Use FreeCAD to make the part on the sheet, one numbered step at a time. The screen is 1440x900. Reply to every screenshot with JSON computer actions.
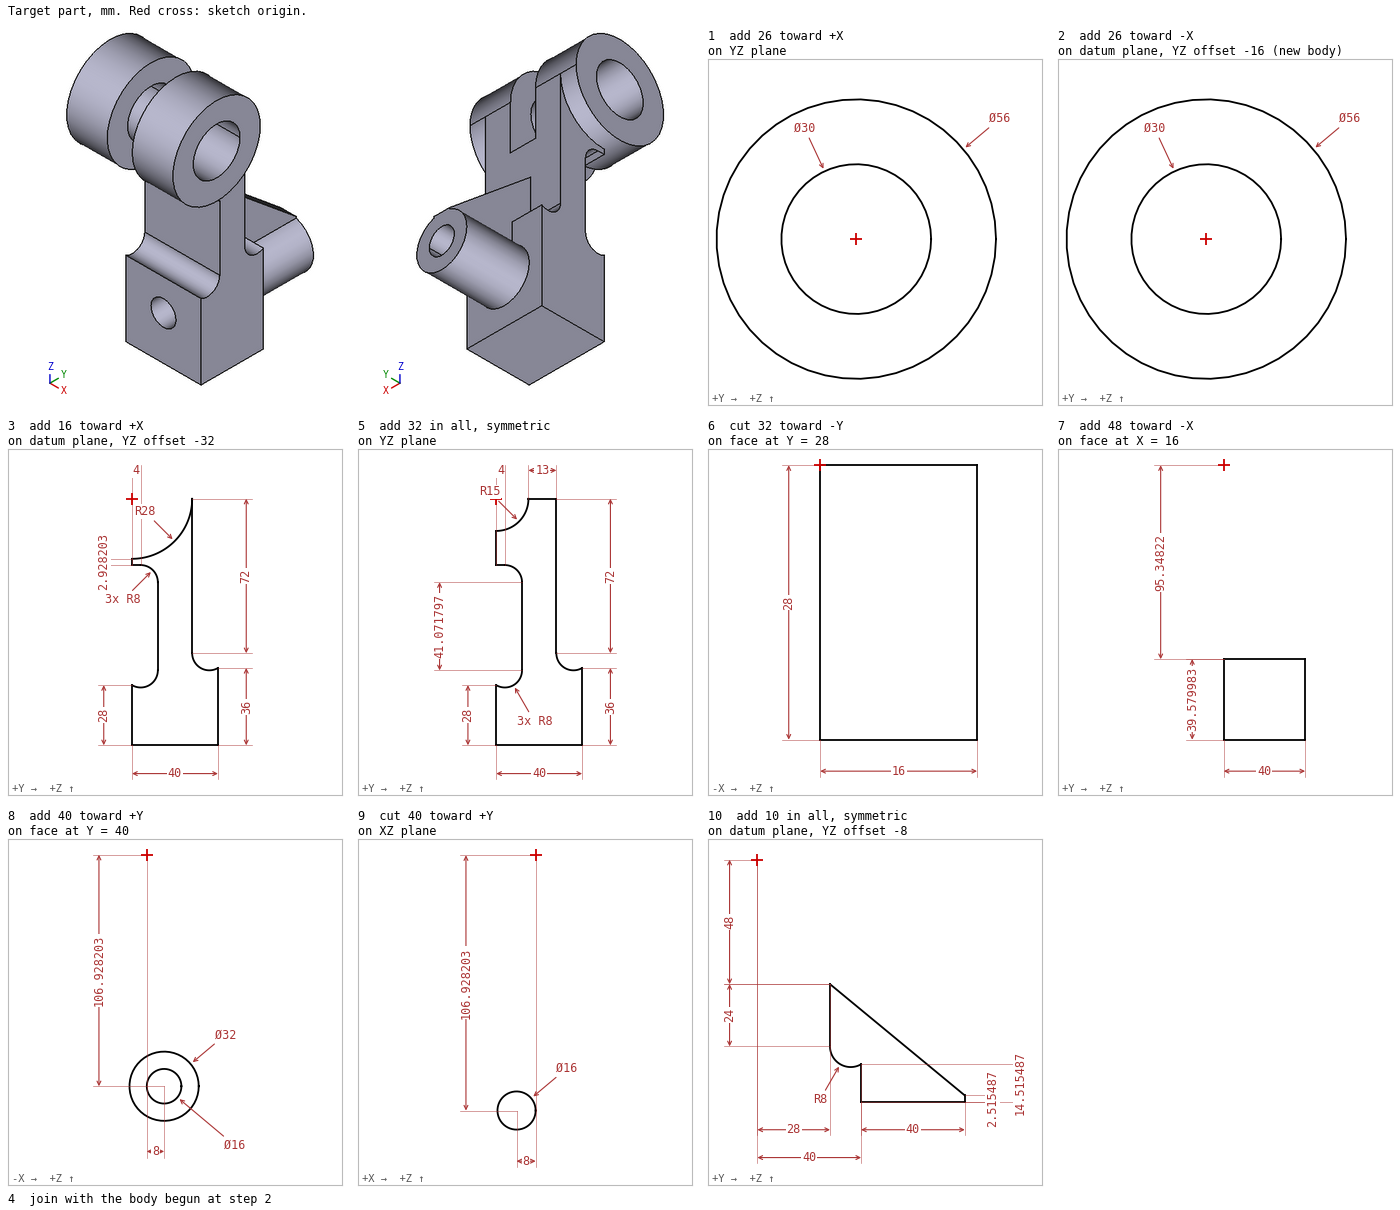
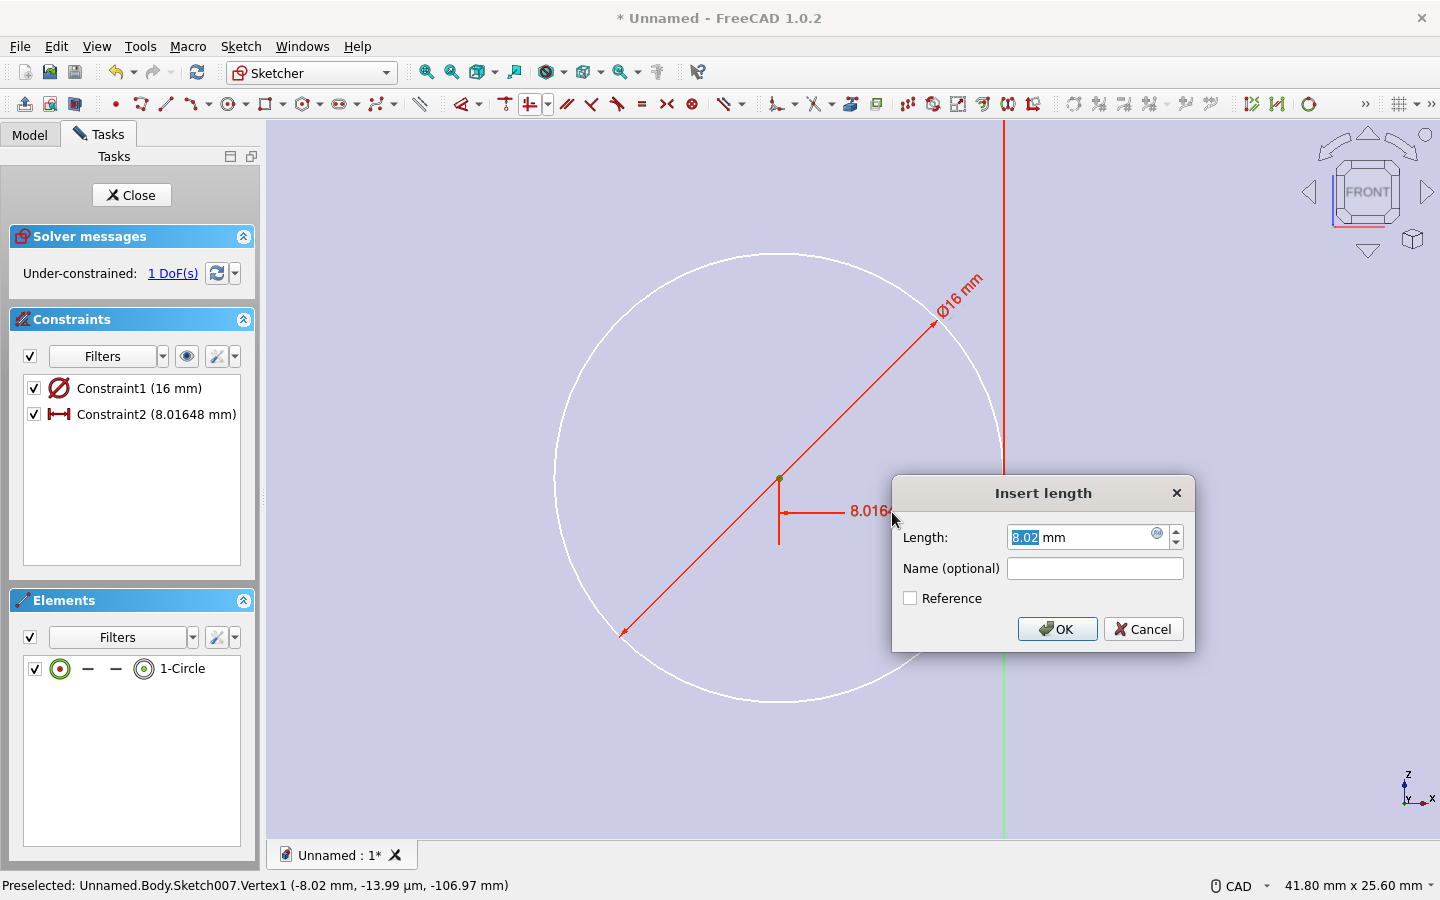
{"action": "type", "text": "8"}
{"action": "key", "text": "Return"}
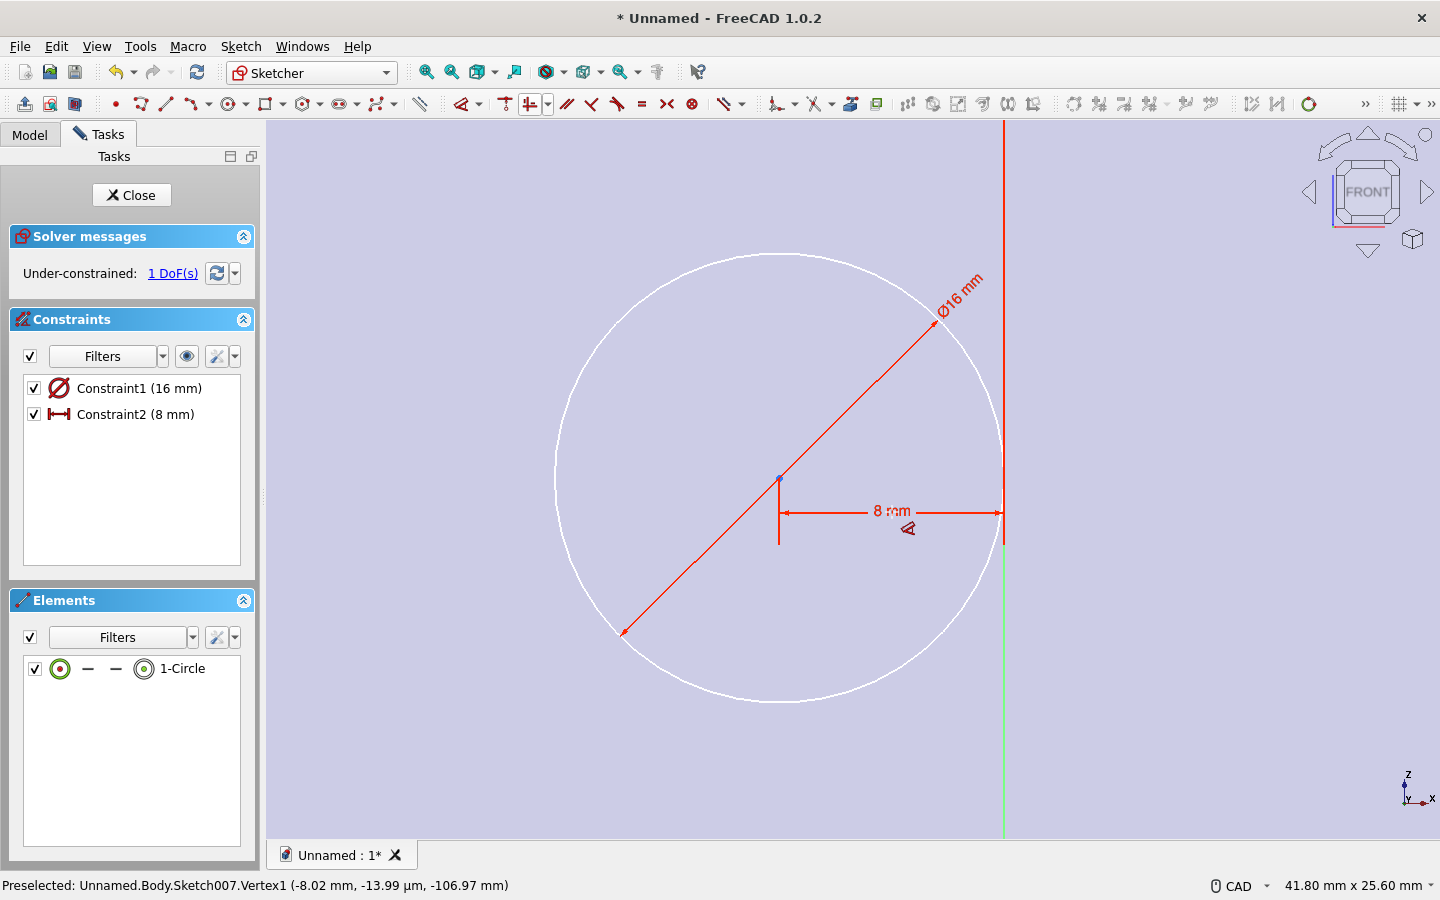
{"action": "left_click", "coordinate": [779, 478]}
{"action": "left_click", "coordinate": [1038, 313]}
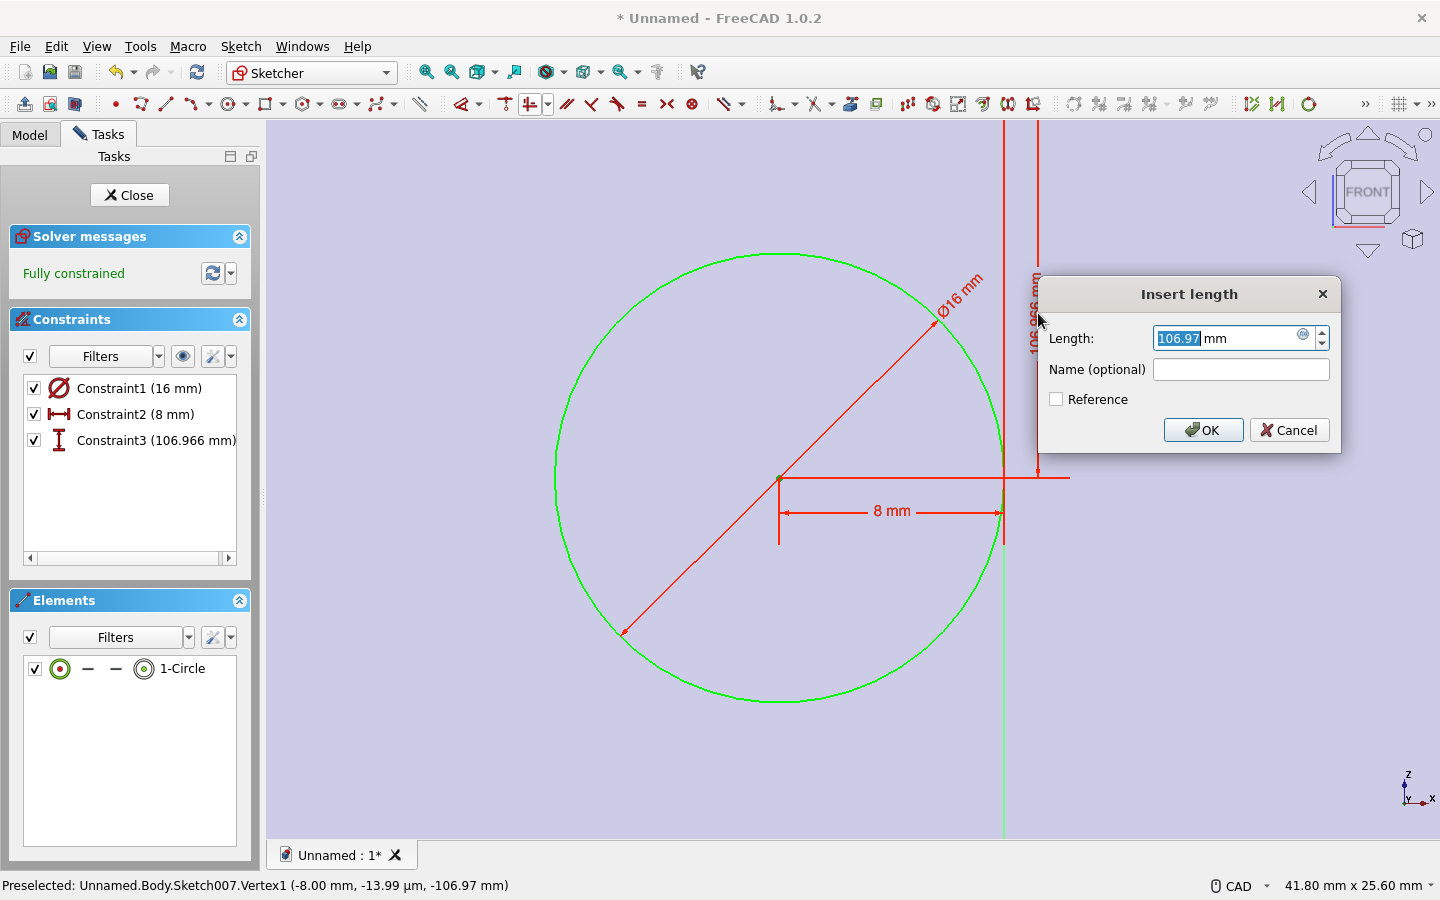
{"action": "type", "text": "106.928203"}
{"action": "key", "text": "Return"}
{"action": "key", "text": "Escape"}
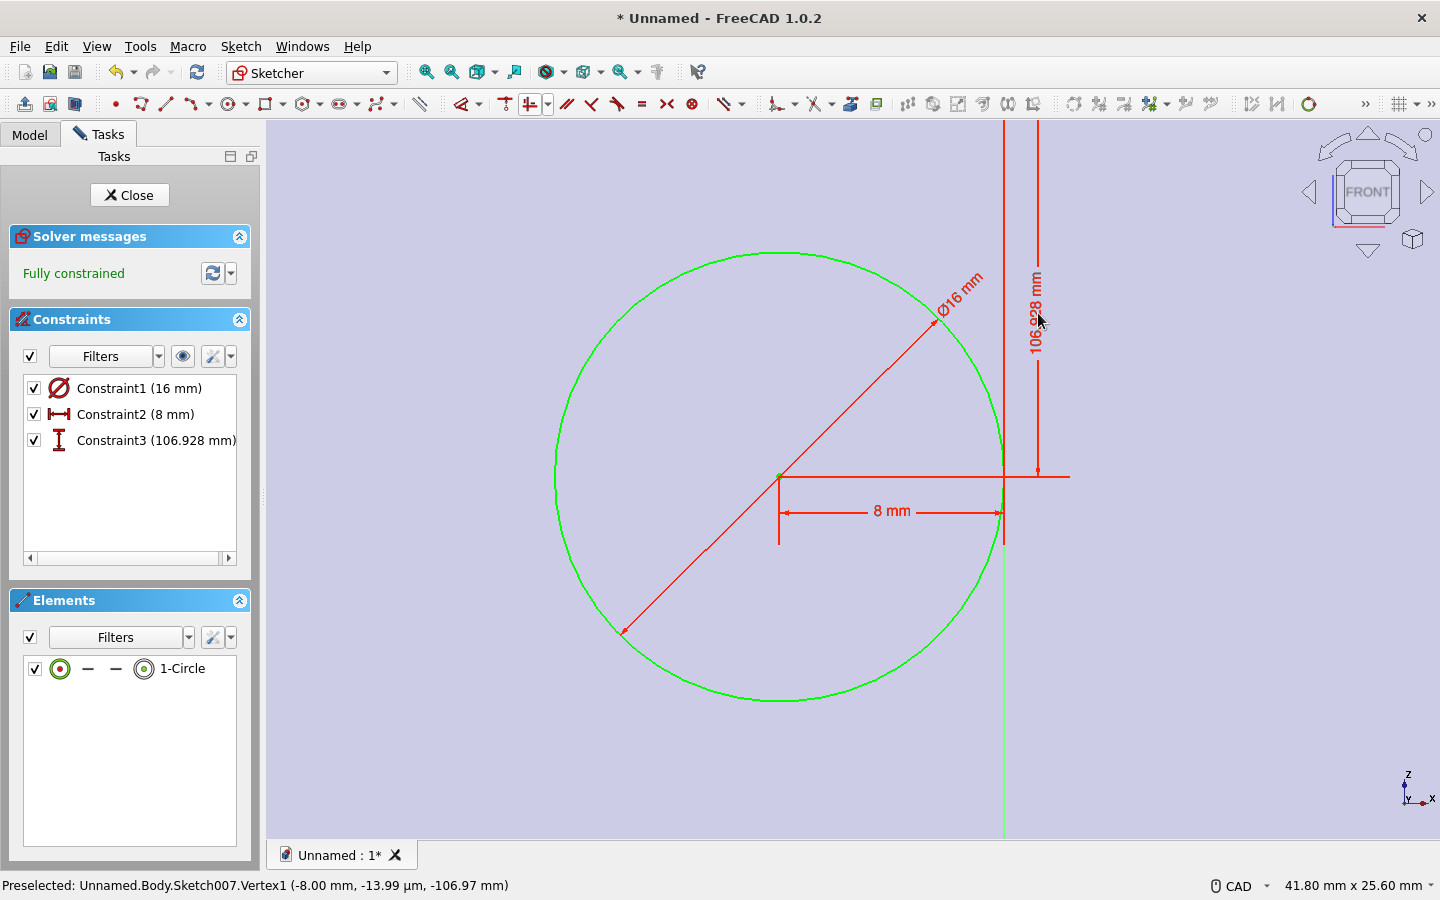
{"action": "left_click", "coordinate": [130, 195]}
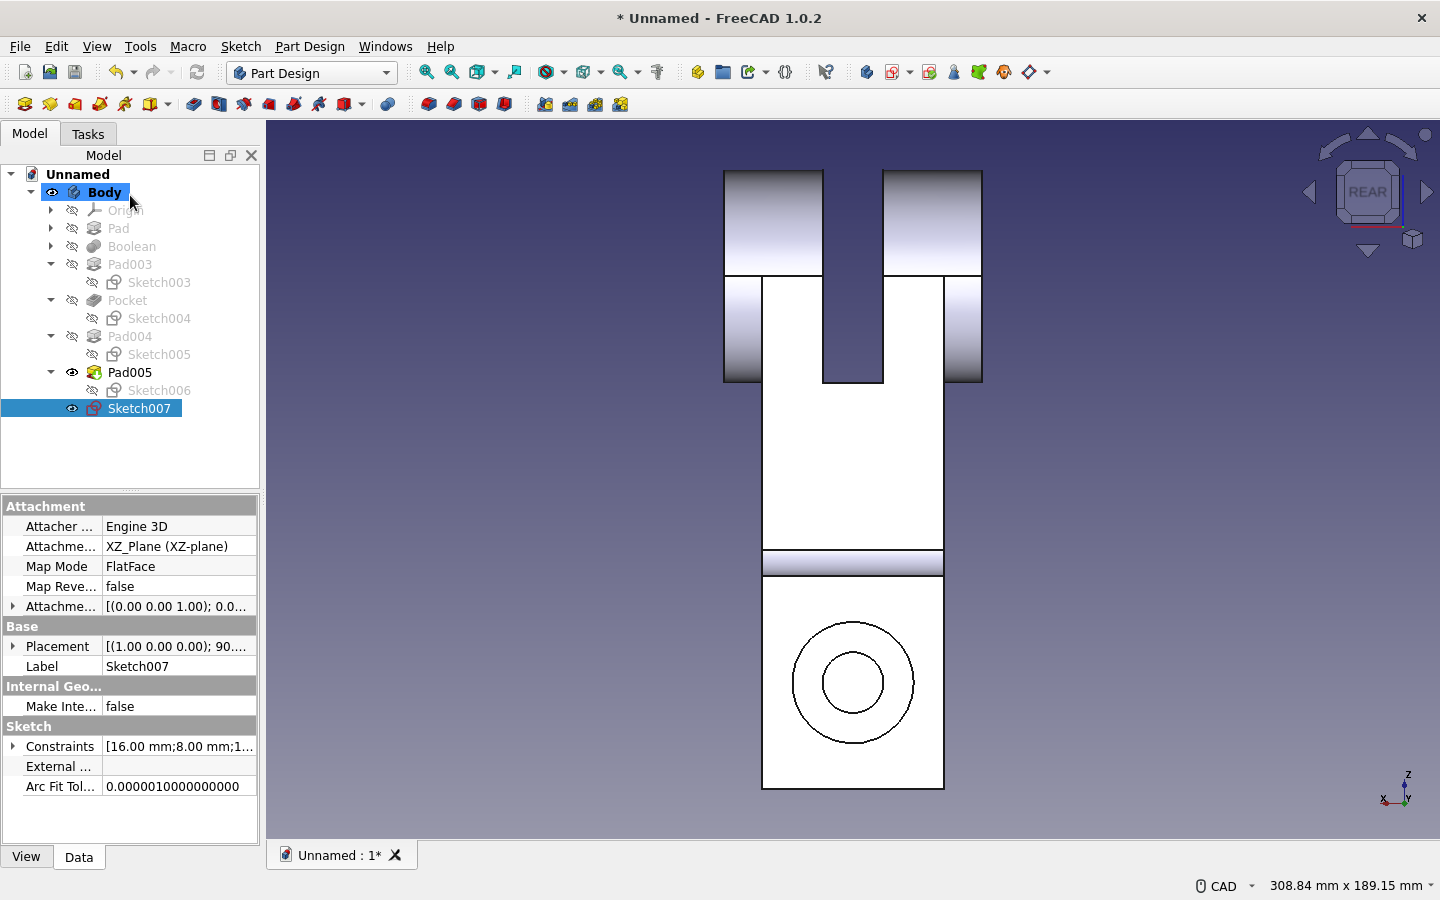
{"action": "left_click", "coordinate": [194, 104]}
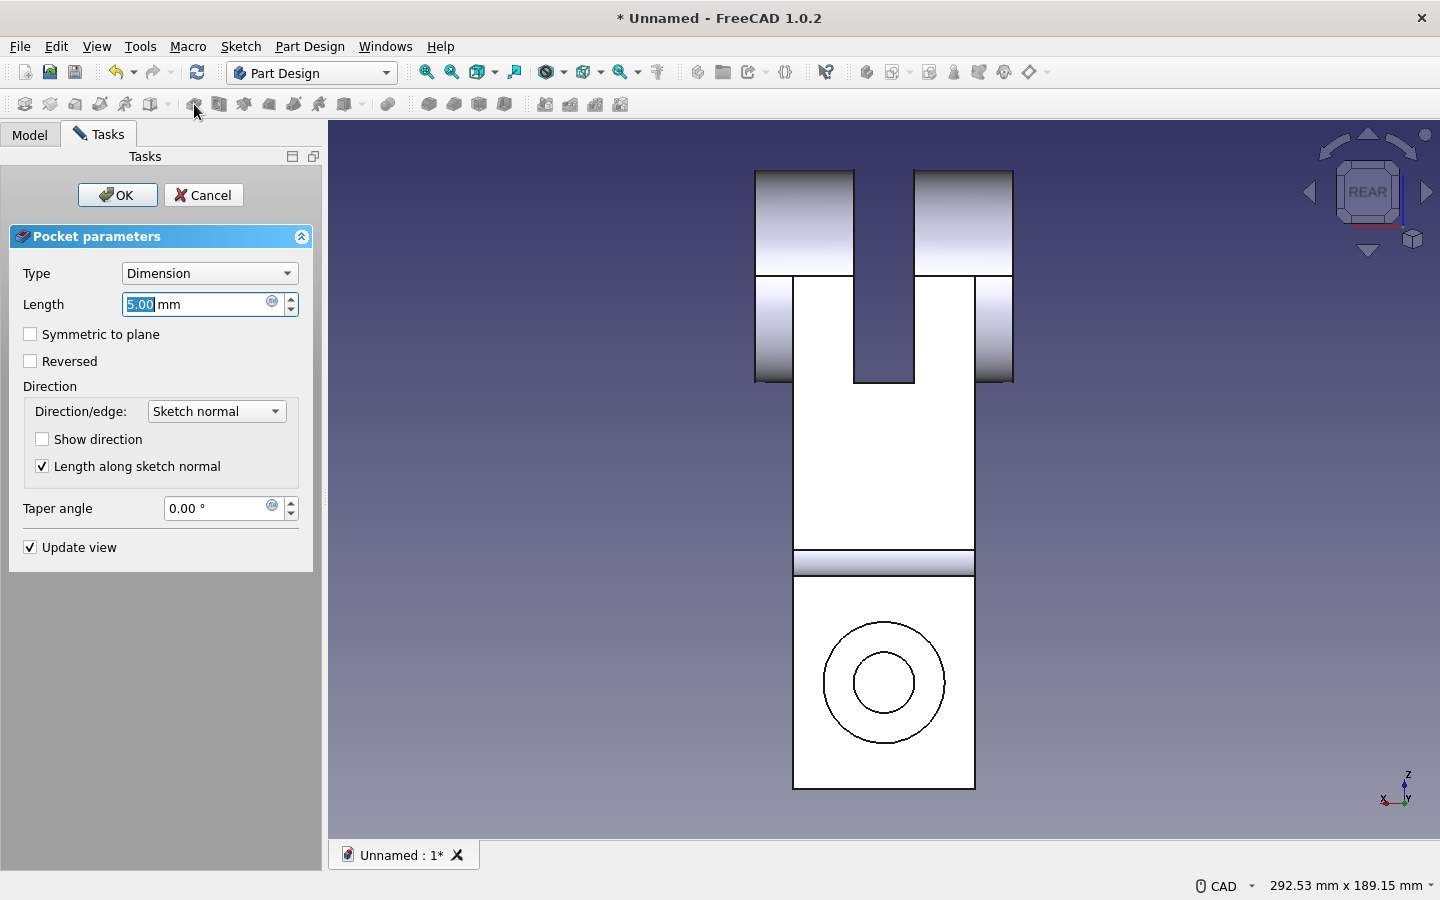
{"action": "type", "text": "40"}
{"action": "key", "text": "Tab"}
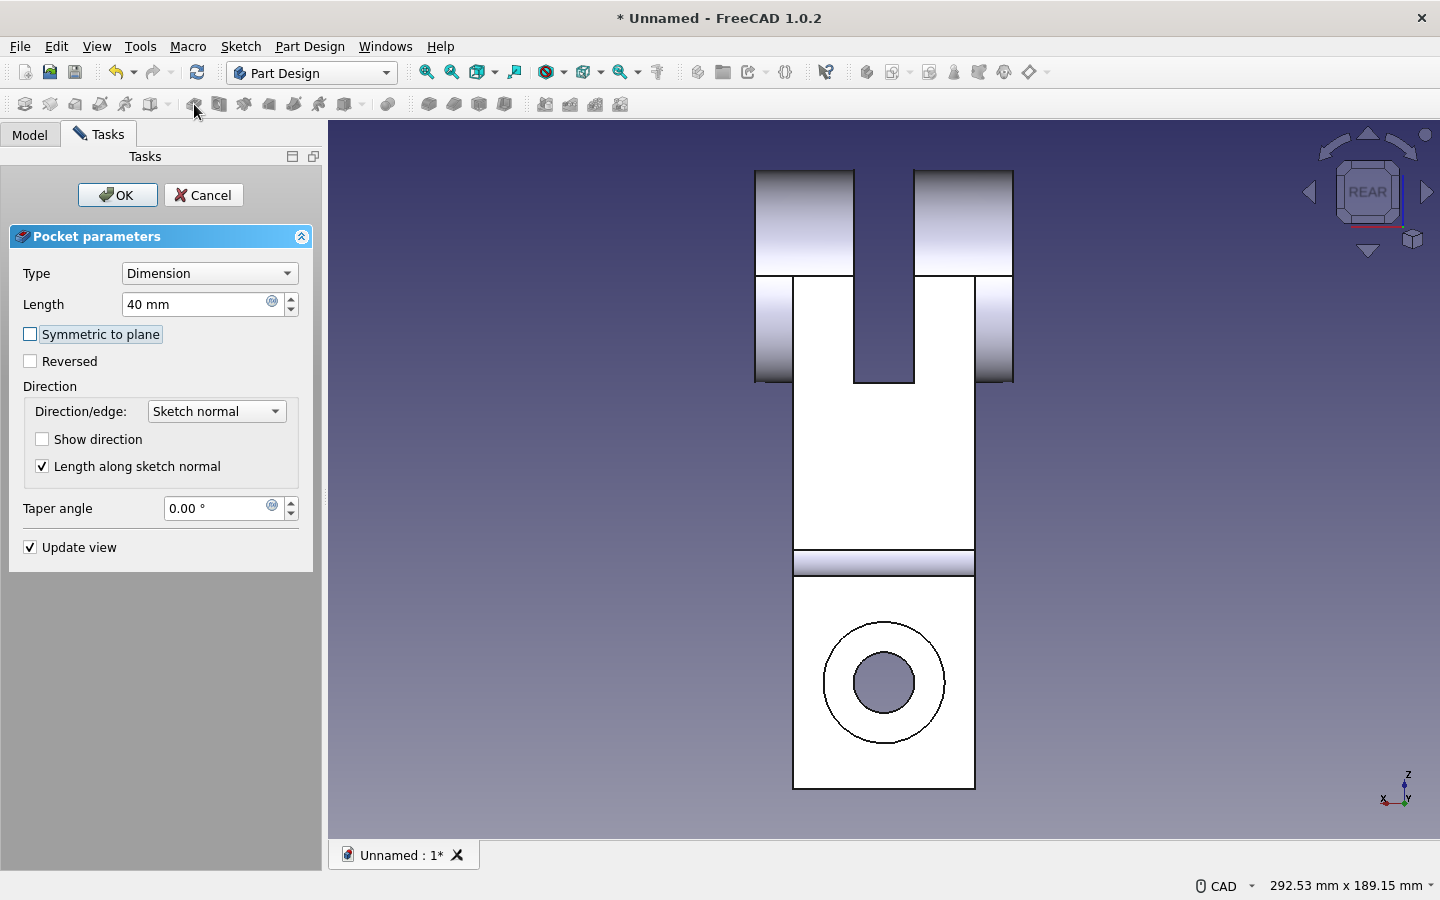
{"action": "left_click", "coordinate": [118, 195]}